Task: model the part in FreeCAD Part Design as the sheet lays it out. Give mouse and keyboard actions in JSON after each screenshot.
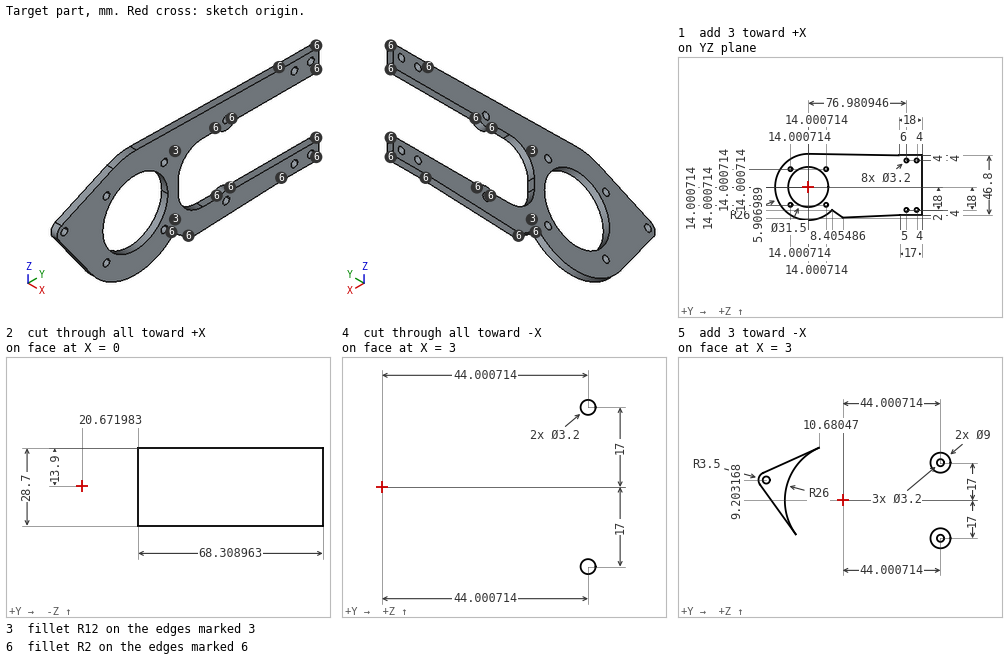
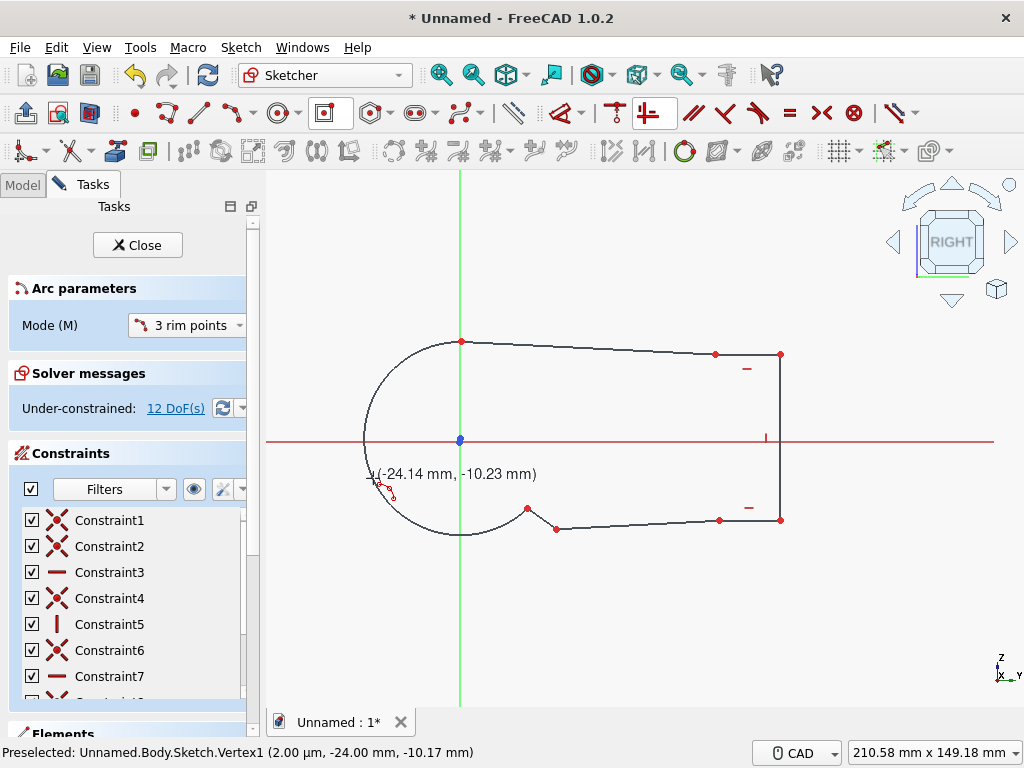
{"action": "left_click", "coordinate": [278, 114]}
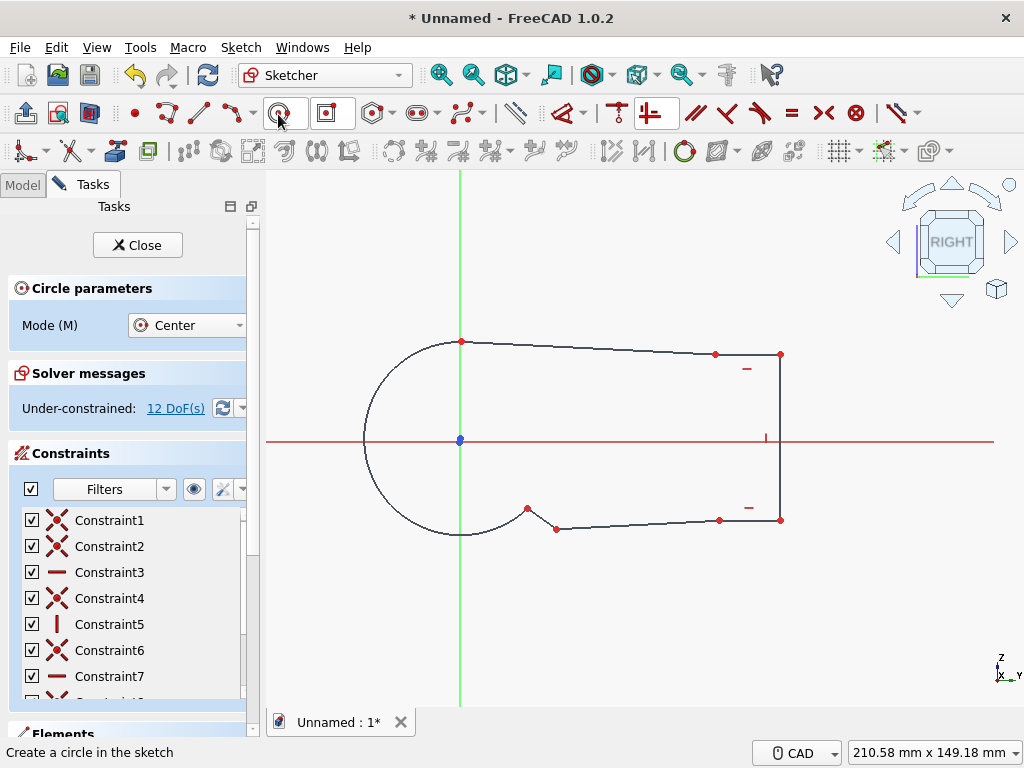
{"action": "scroll", "coordinate": [409, 392], "scroll_direction": "up", "scroll_amount": 7}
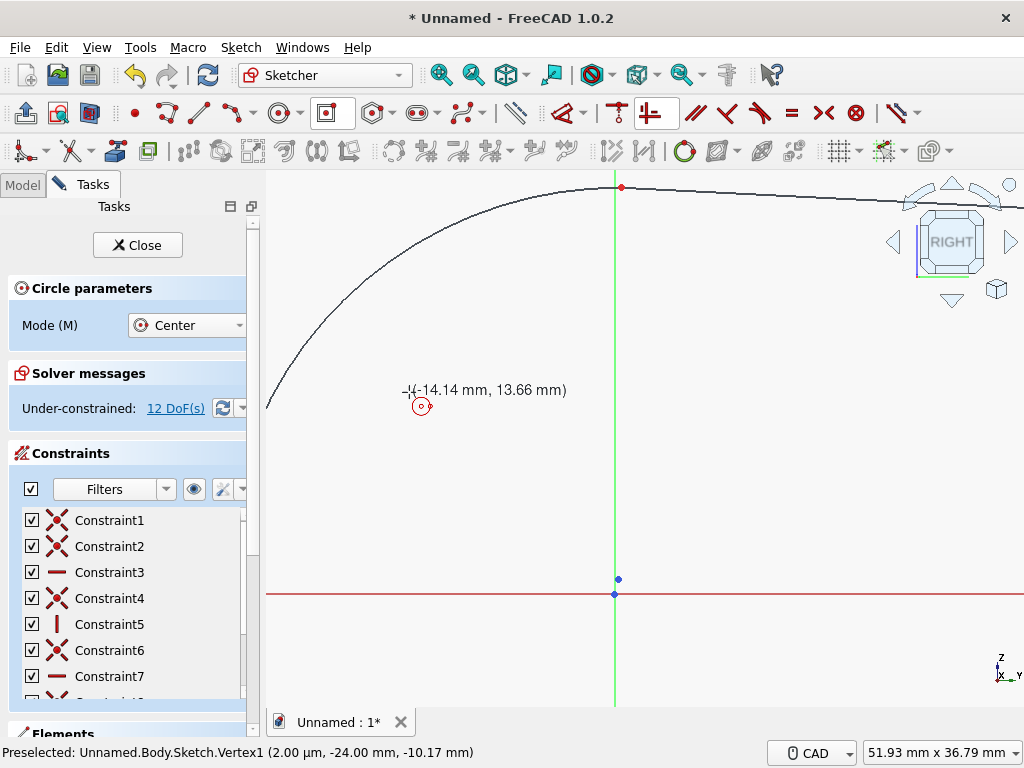
{"action": "scroll", "coordinate": [409, 392], "scroll_direction": "down", "scroll_amount": 7}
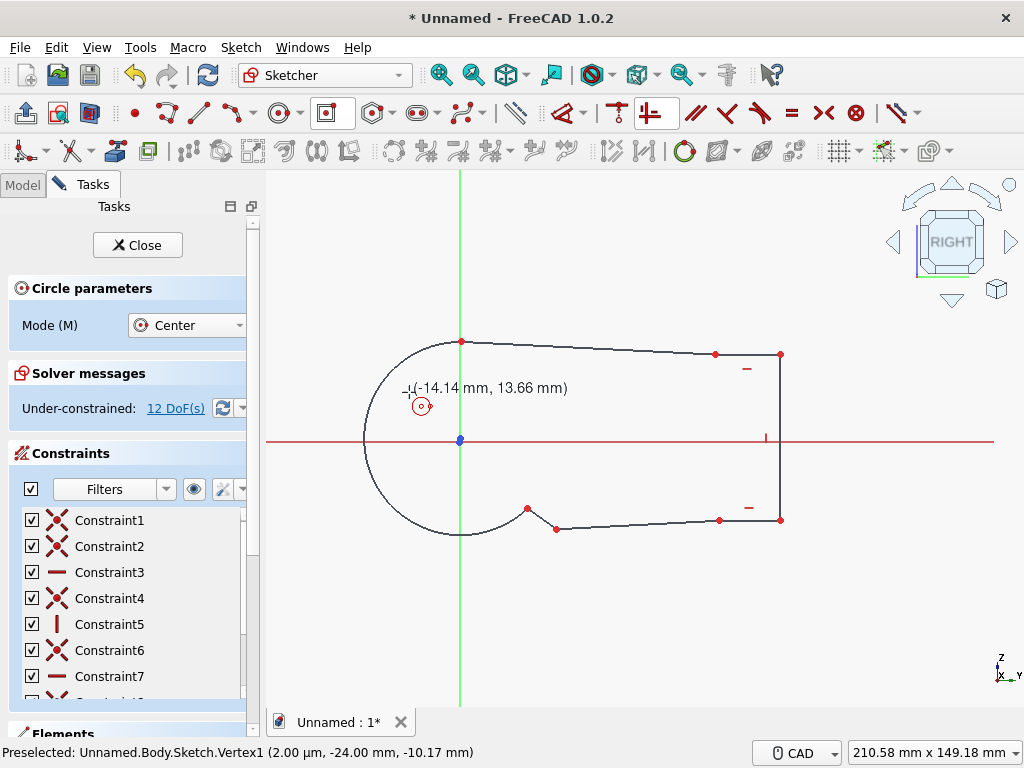
{"action": "left_click", "coordinate": [409, 392]}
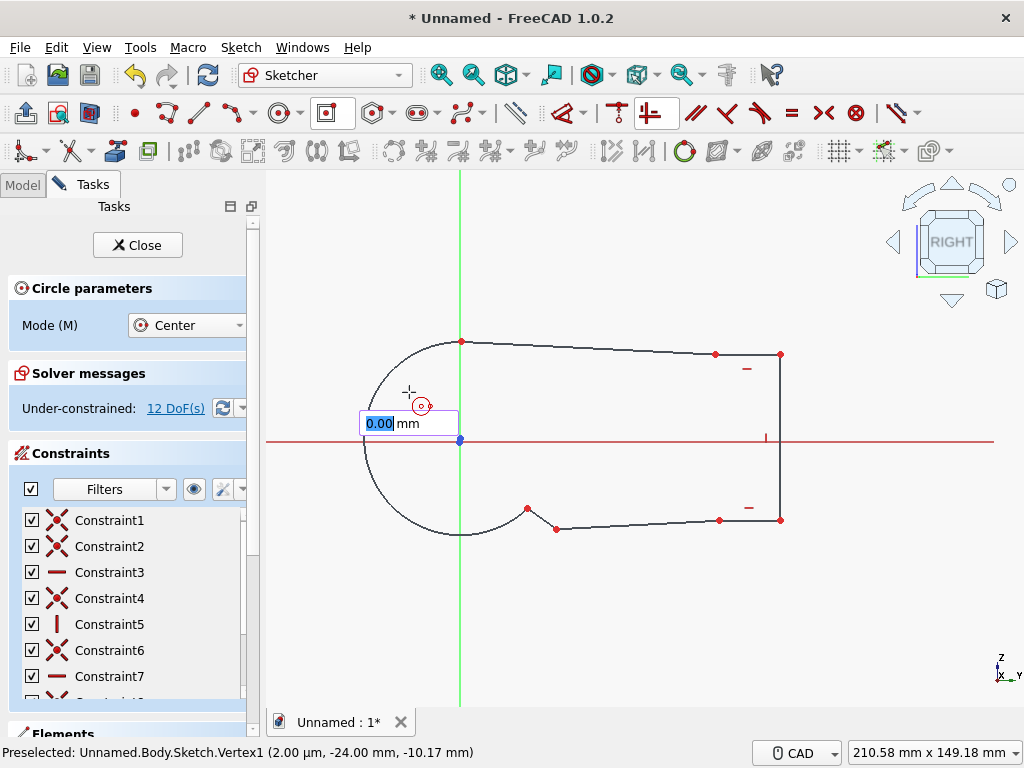
{"action": "scroll", "coordinate": [414, 388], "scroll_direction": "up", "scroll_amount": 6}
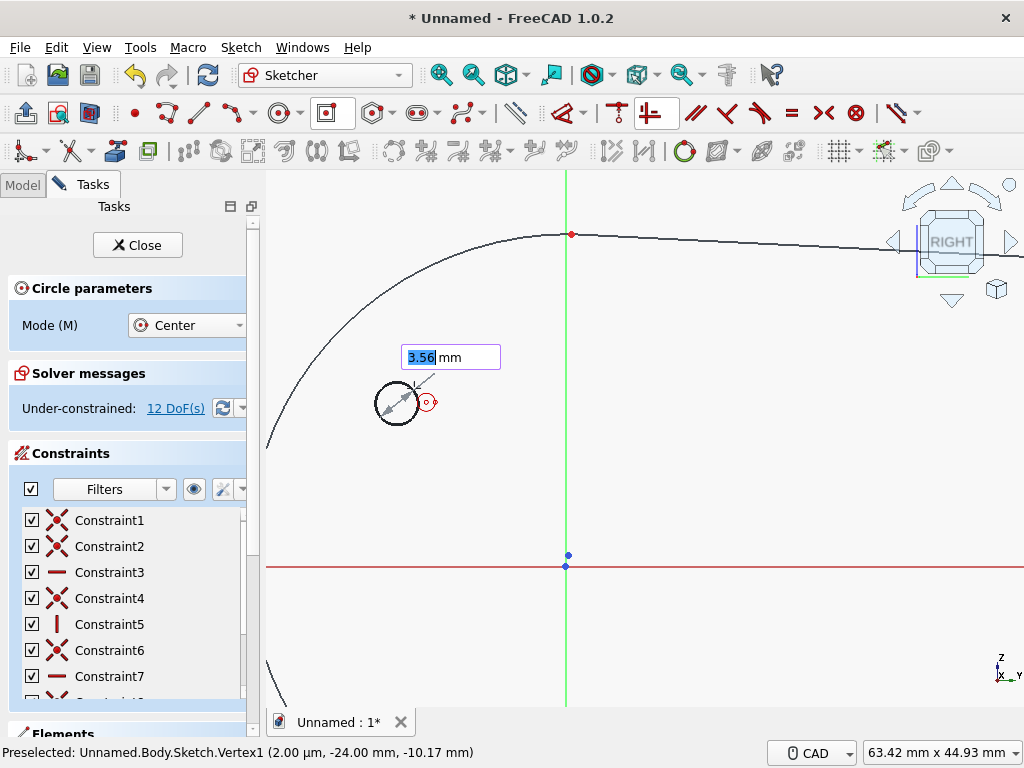
{"action": "left_click", "coordinate": [412, 386]}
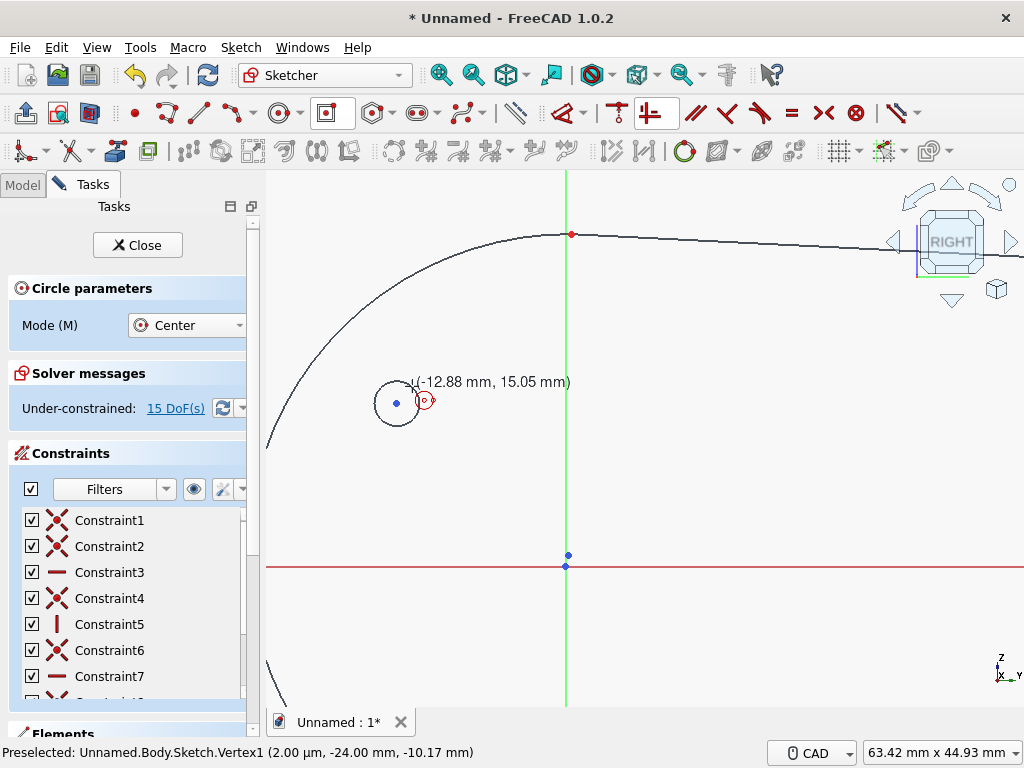
{"action": "scroll", "coordinate": [414, 388], "scroll_direction": "down", "scroll_amount": 6}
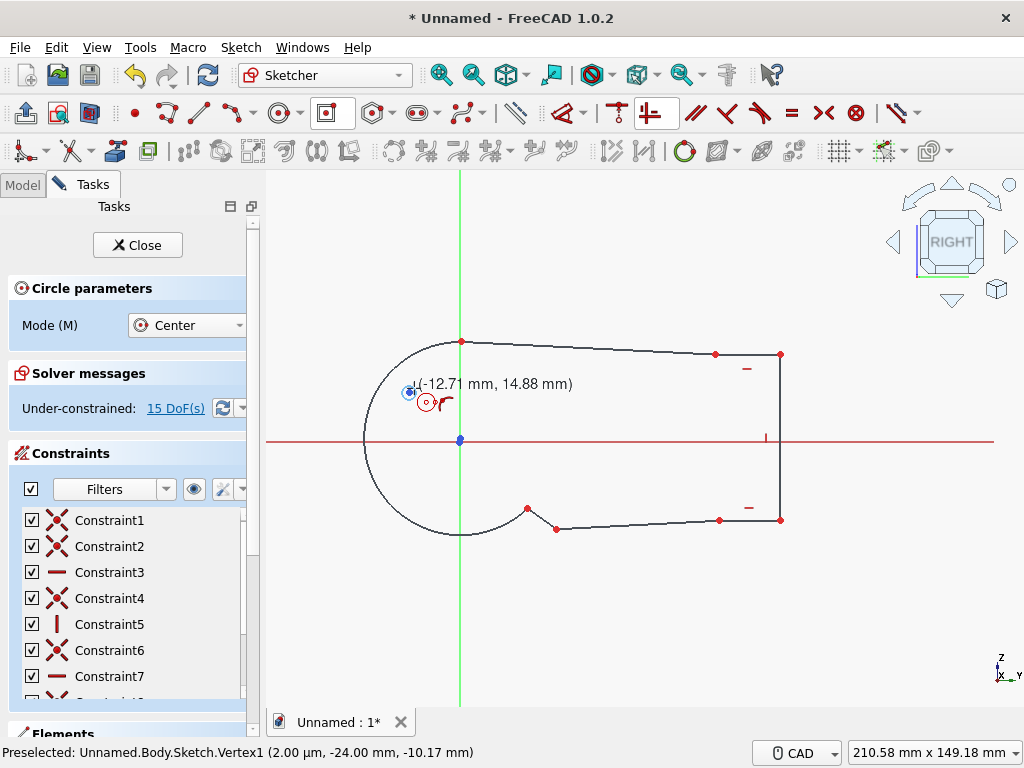
{"action": "left_click", "coordinate": [510, 392]}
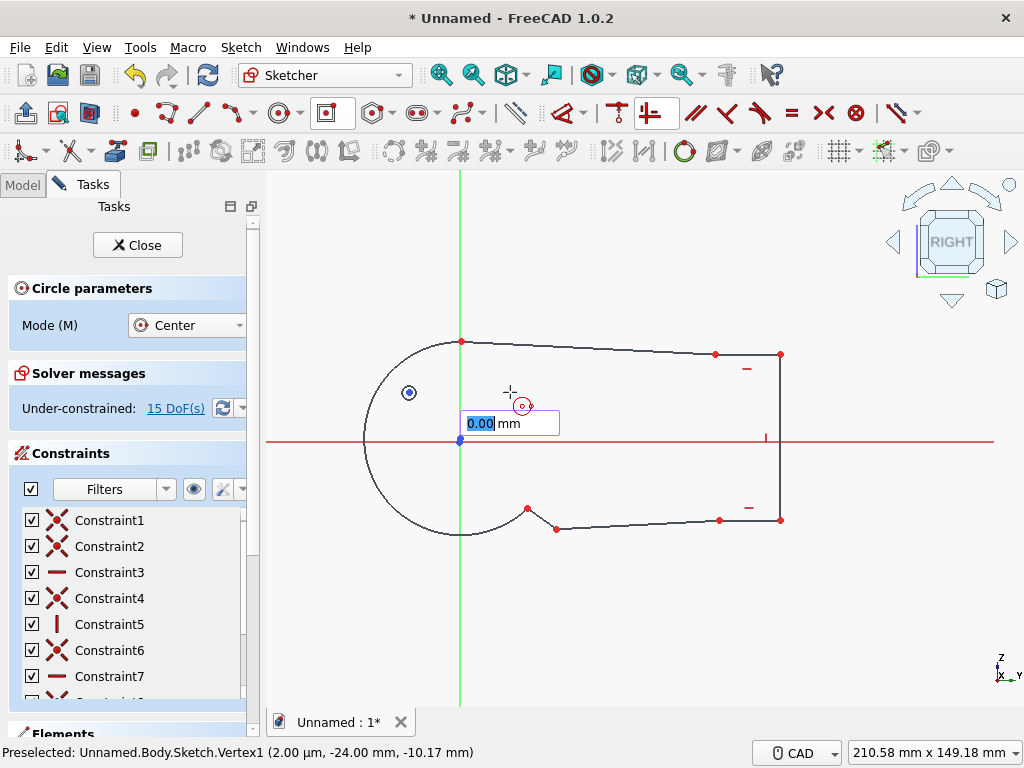
{"action": "scroll", "coordinate": [514, 388], "scroll_direction": "up", "scroll_amount": 6}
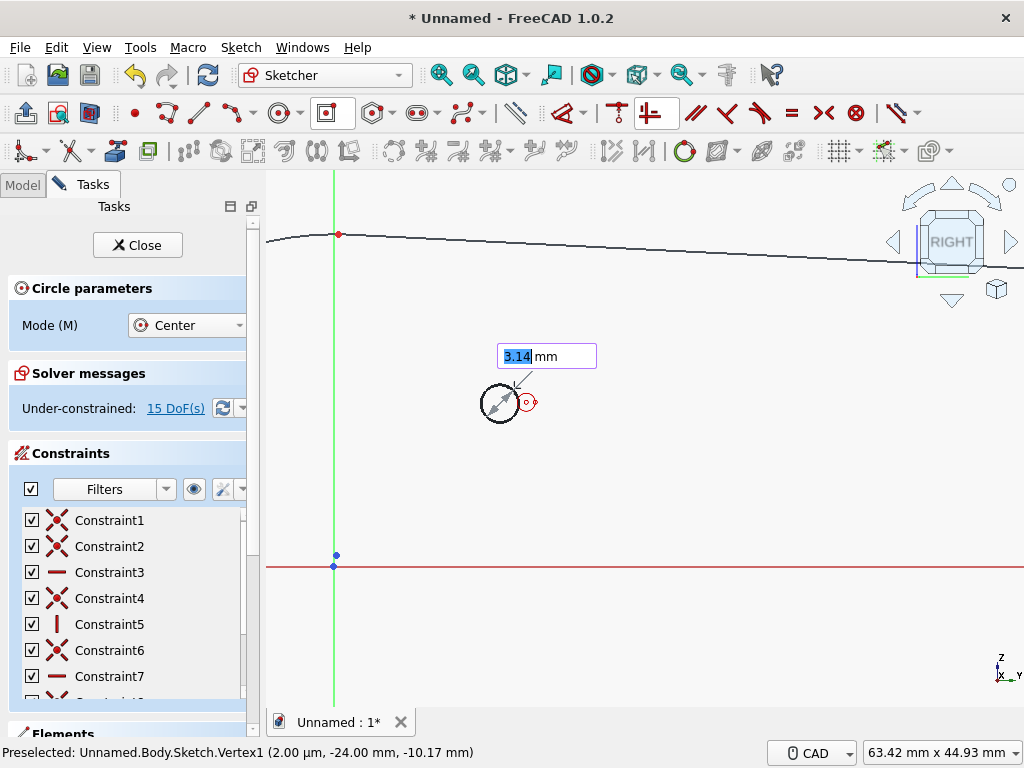
{"action": "left_click", "coordinate": [514, 386]}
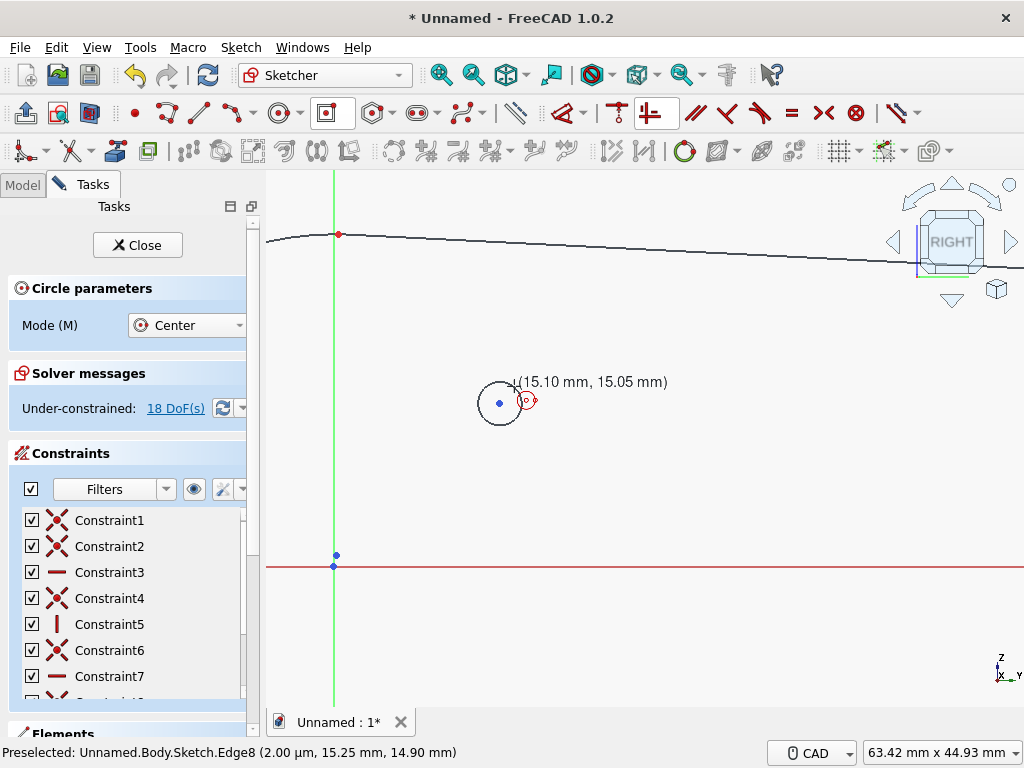
{"action": "scroll", "coordinate": [514, 388], "scroll_direction": "down", "scroll_amount": 6}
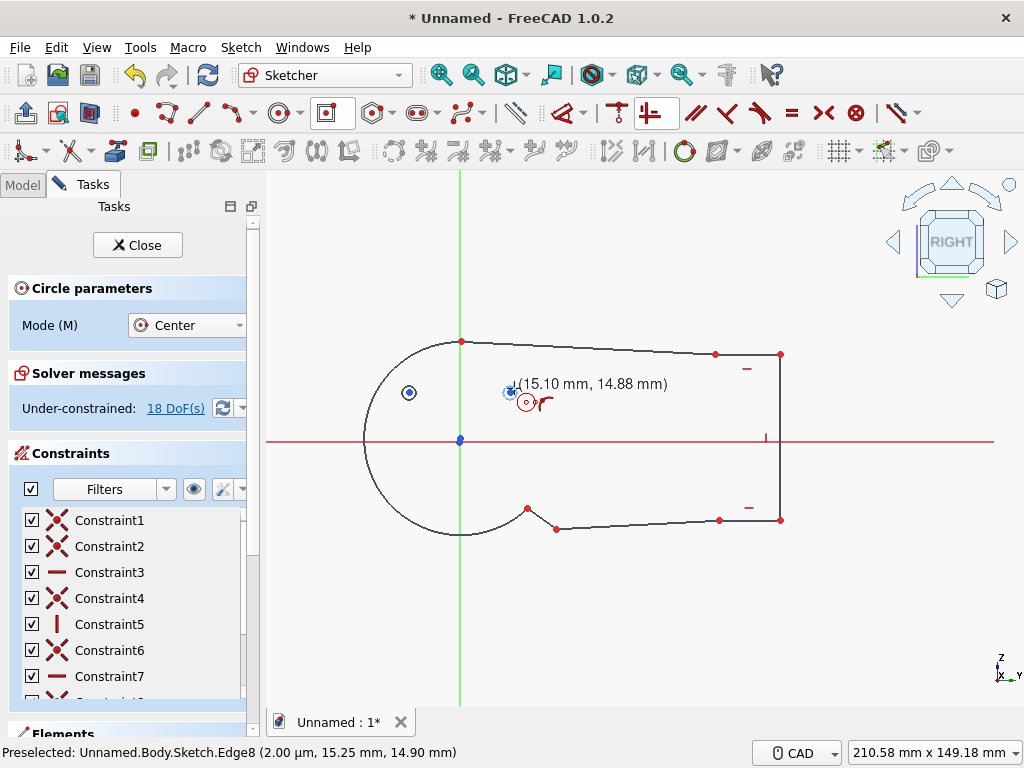
{"action": "left_click", "coordinate": [460, 442]}
{"action": "left_click", "coordinate": [500, 482]}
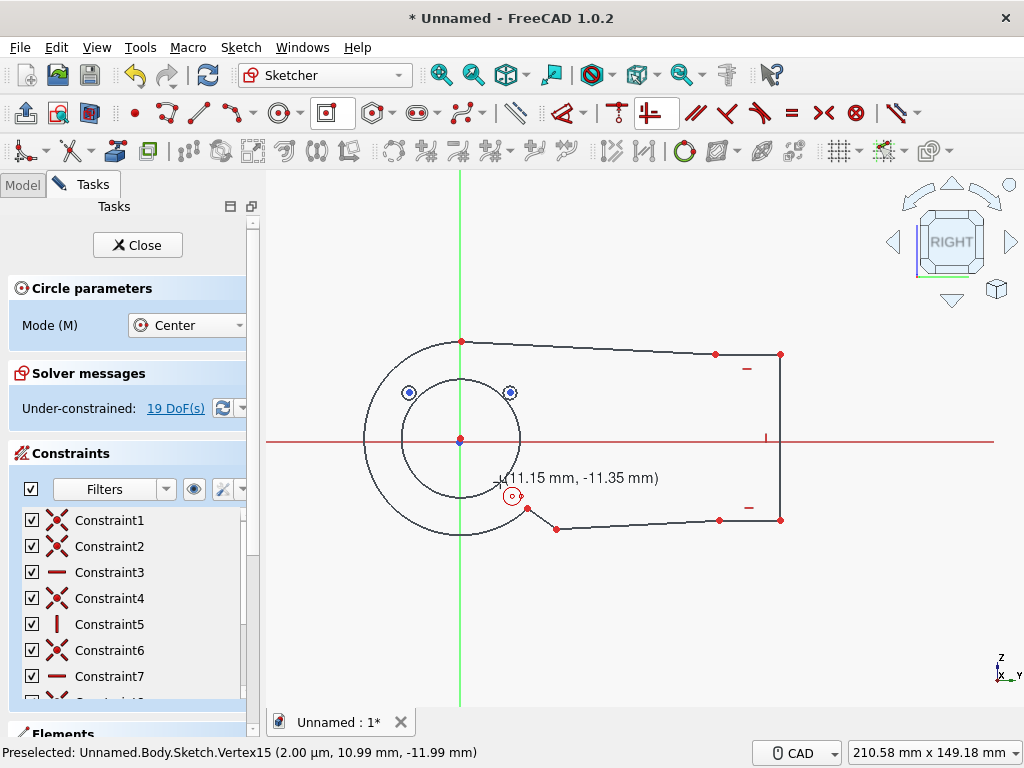
{"action": "scroll", "coordinate": [409, 493], "scroll_direction": "up", "scroll_amount": 7}